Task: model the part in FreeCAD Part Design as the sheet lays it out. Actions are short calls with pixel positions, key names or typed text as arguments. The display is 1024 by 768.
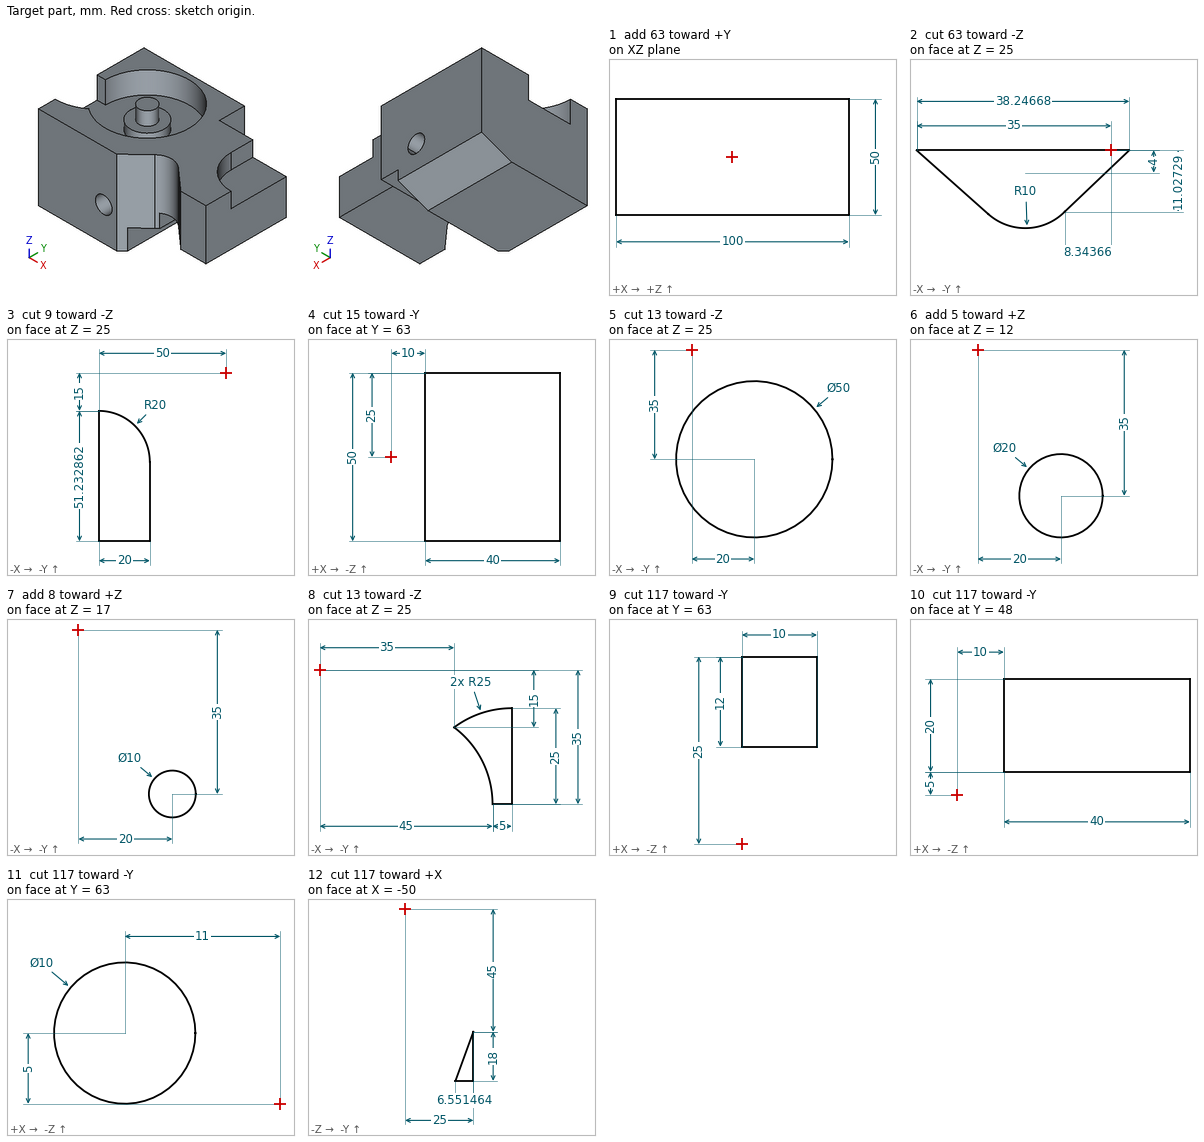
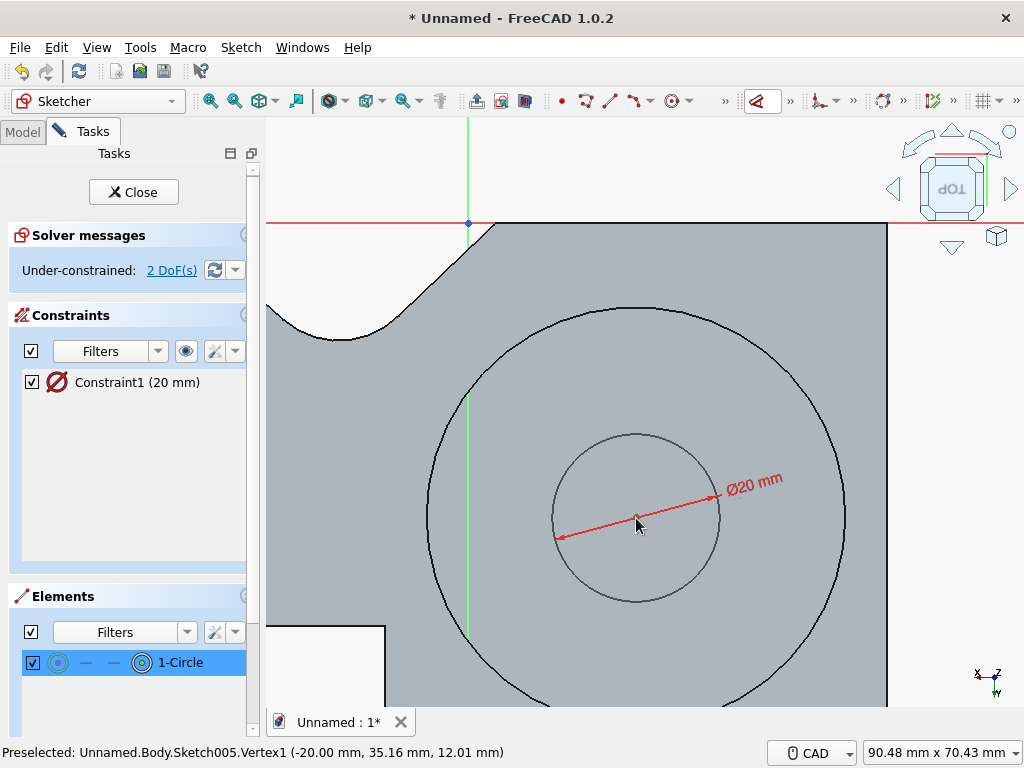
click(776, 102)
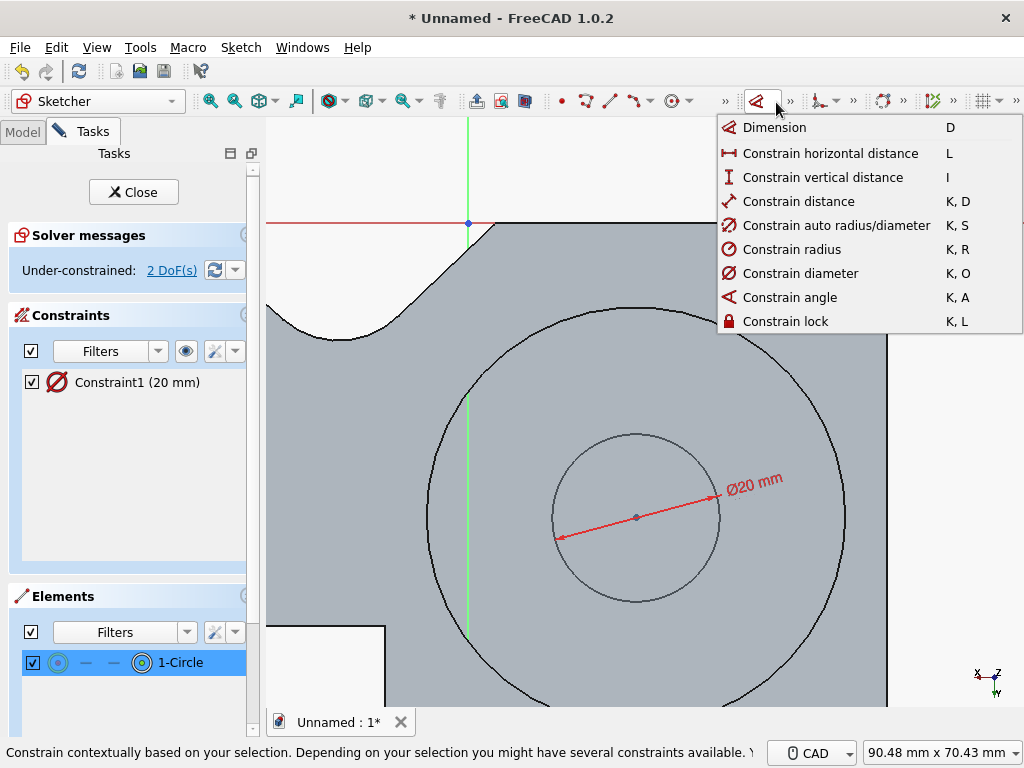
click(870, 153)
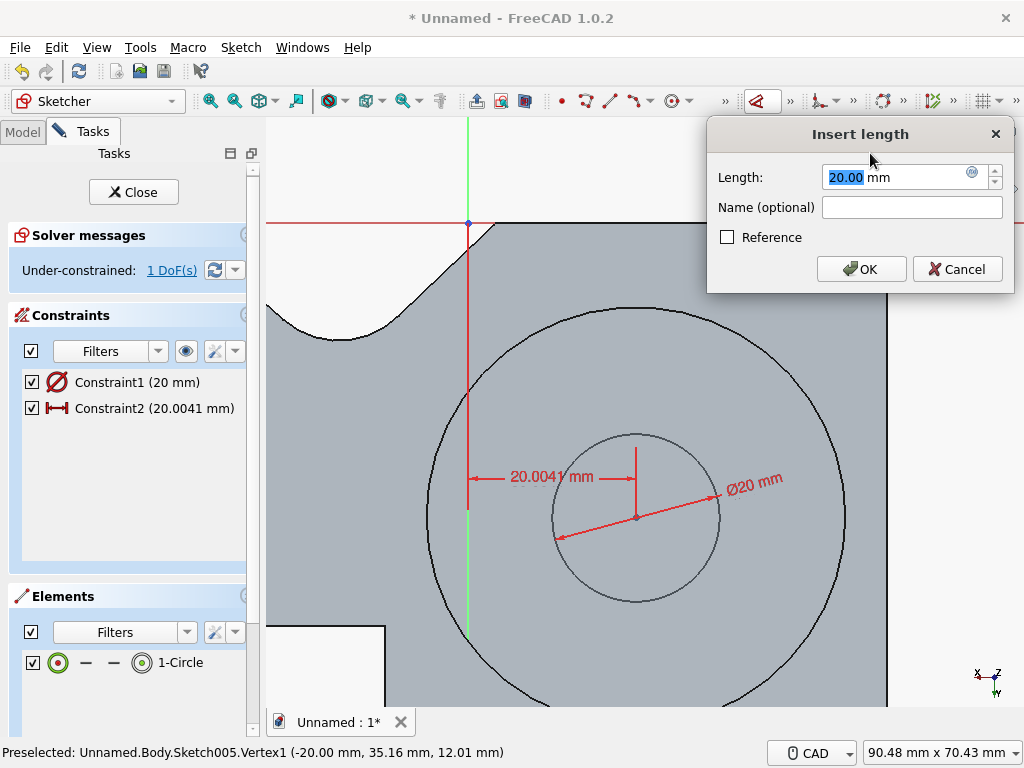
text(20)
key(Return)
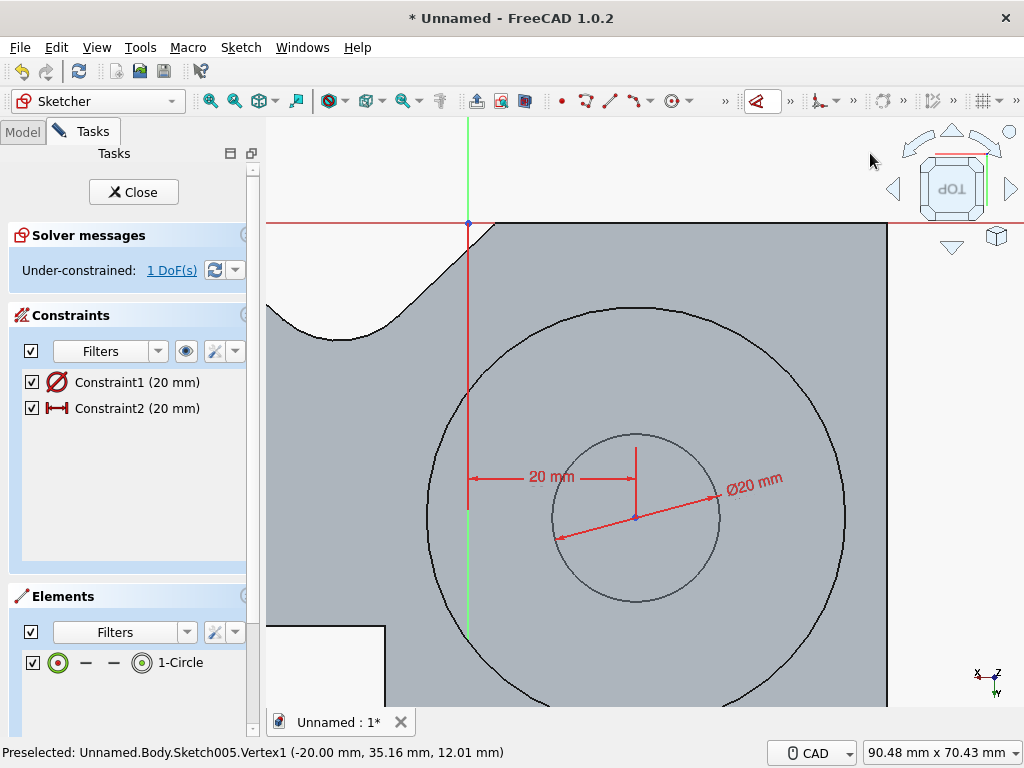
click(636, 518)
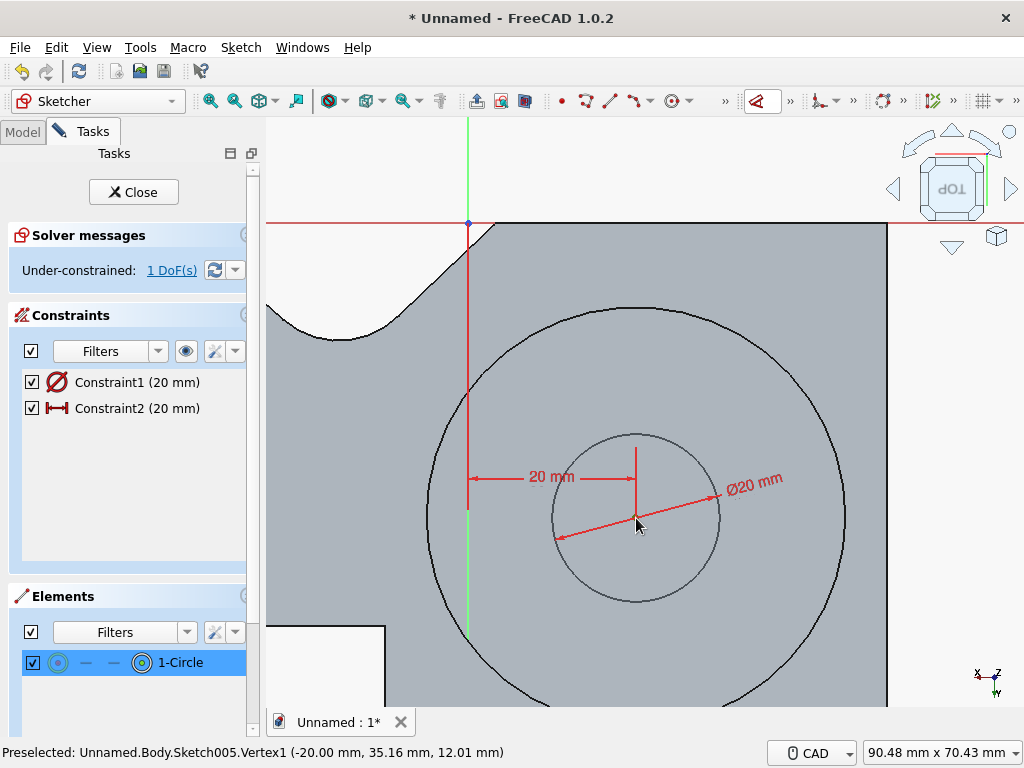
key(i)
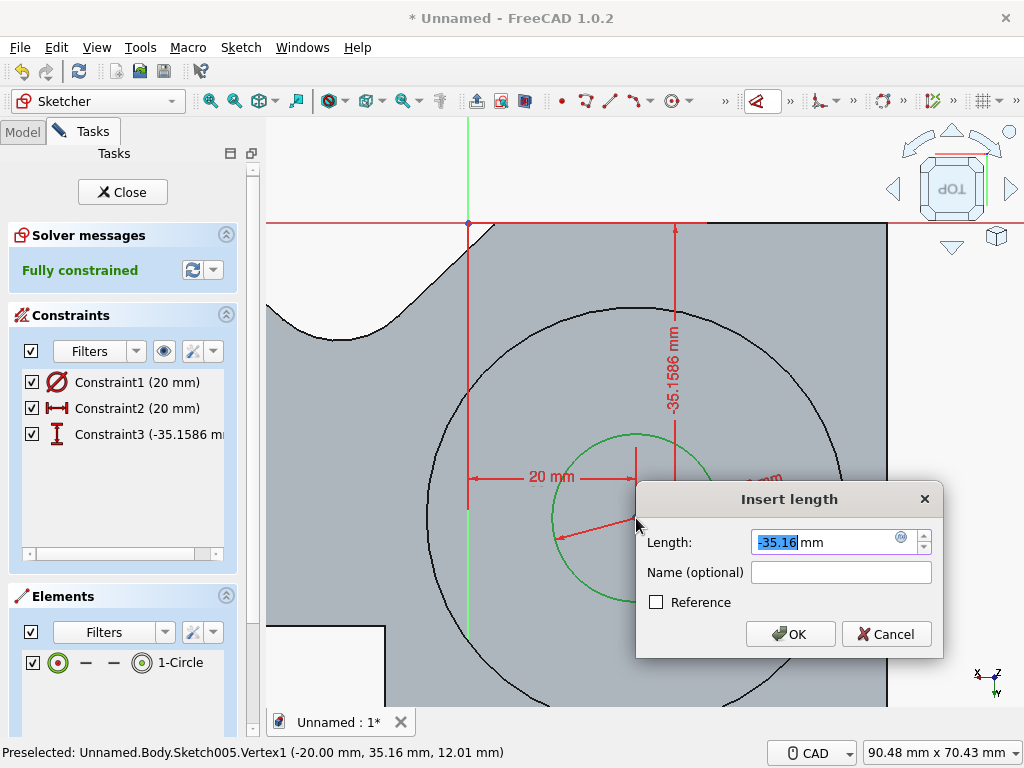
text(-35)
key(Return)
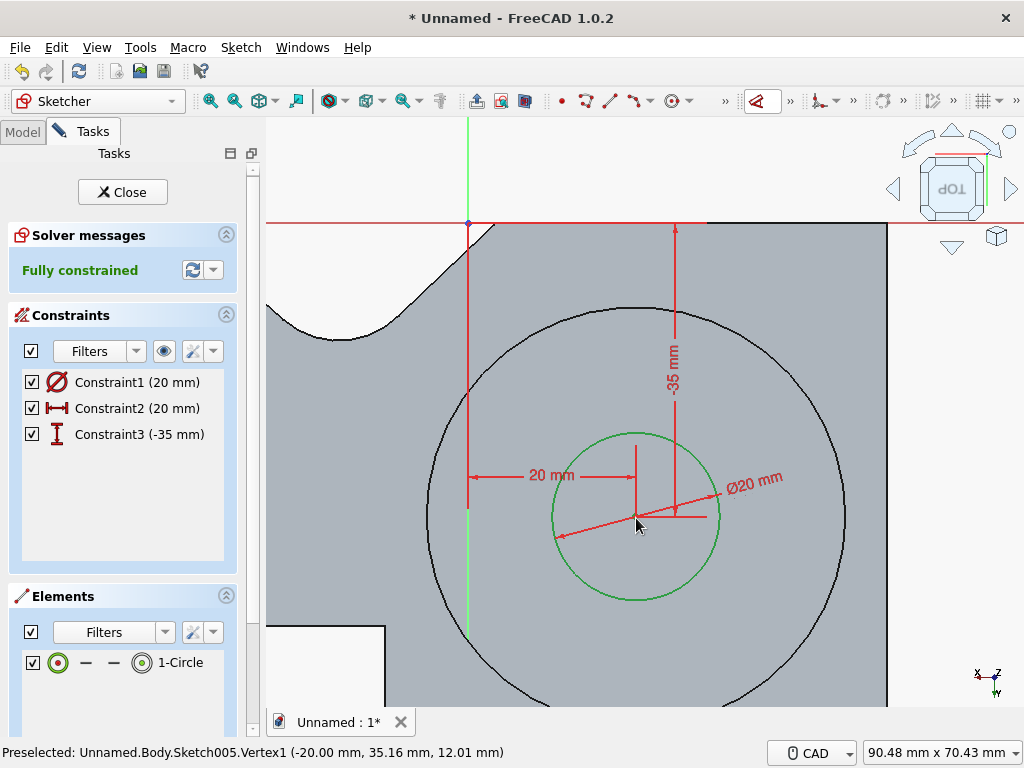
click(123, 192)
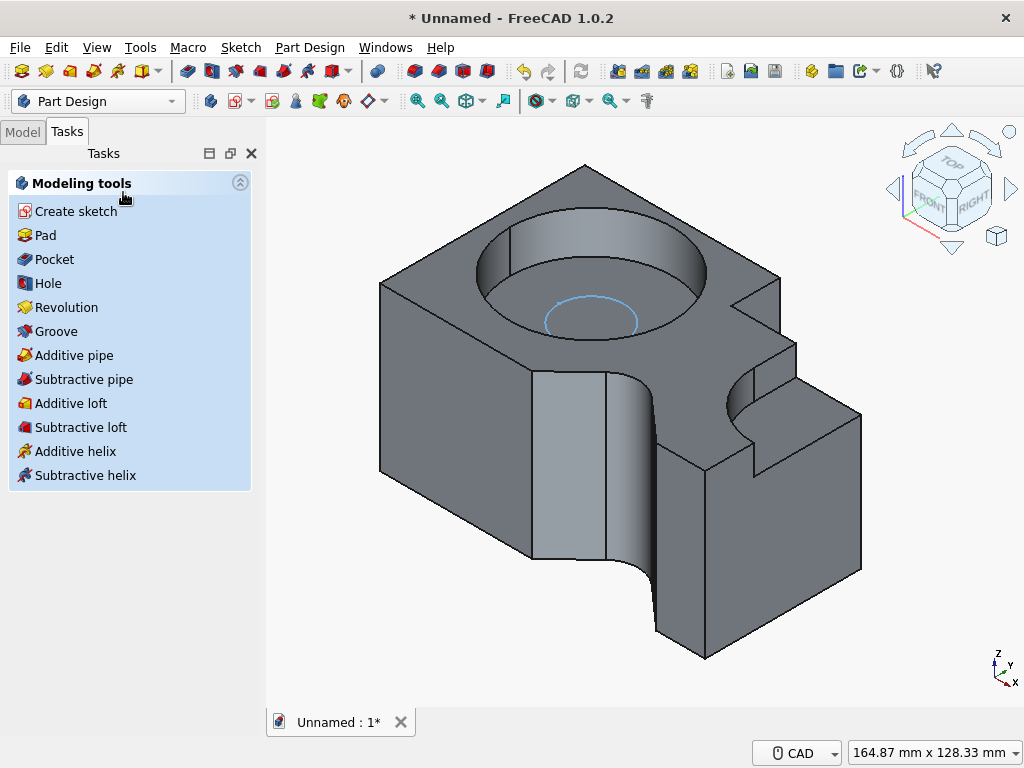
click(22, 72)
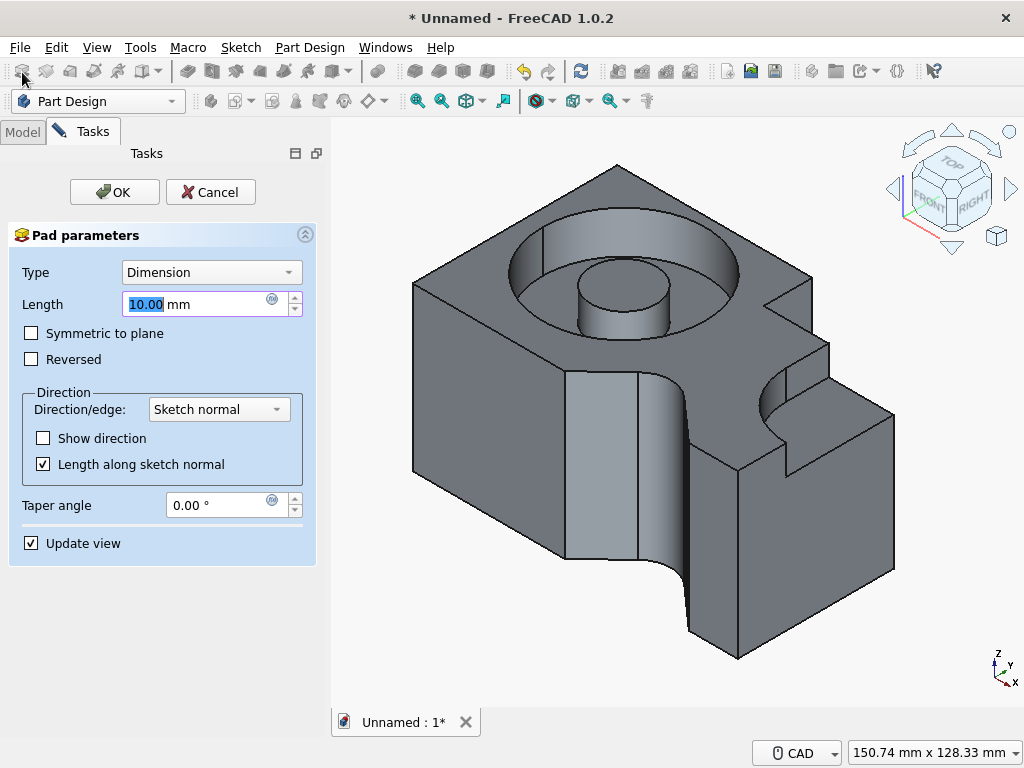
text(5)
key(Tab)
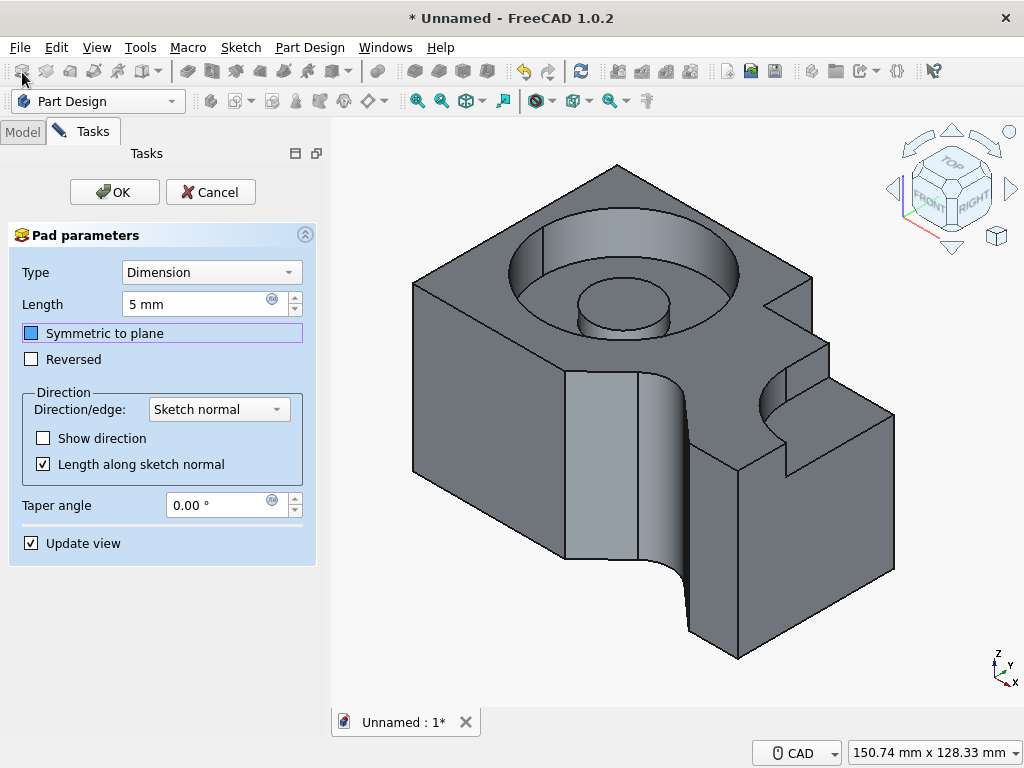
click(115, 192)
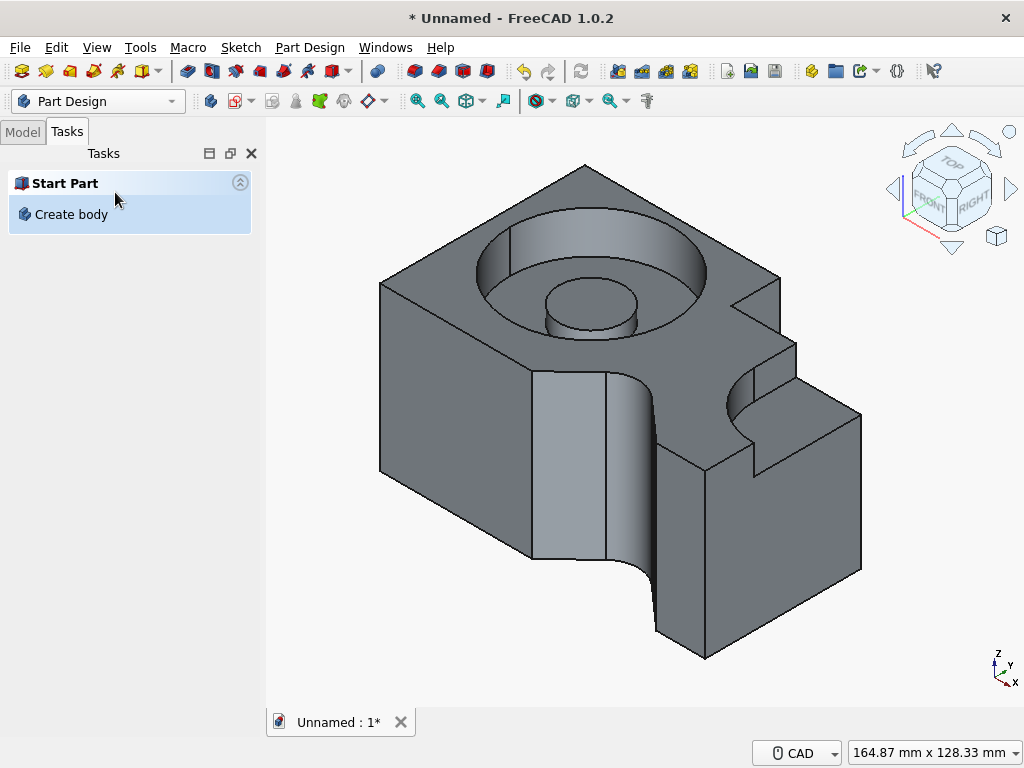
click(591, 303)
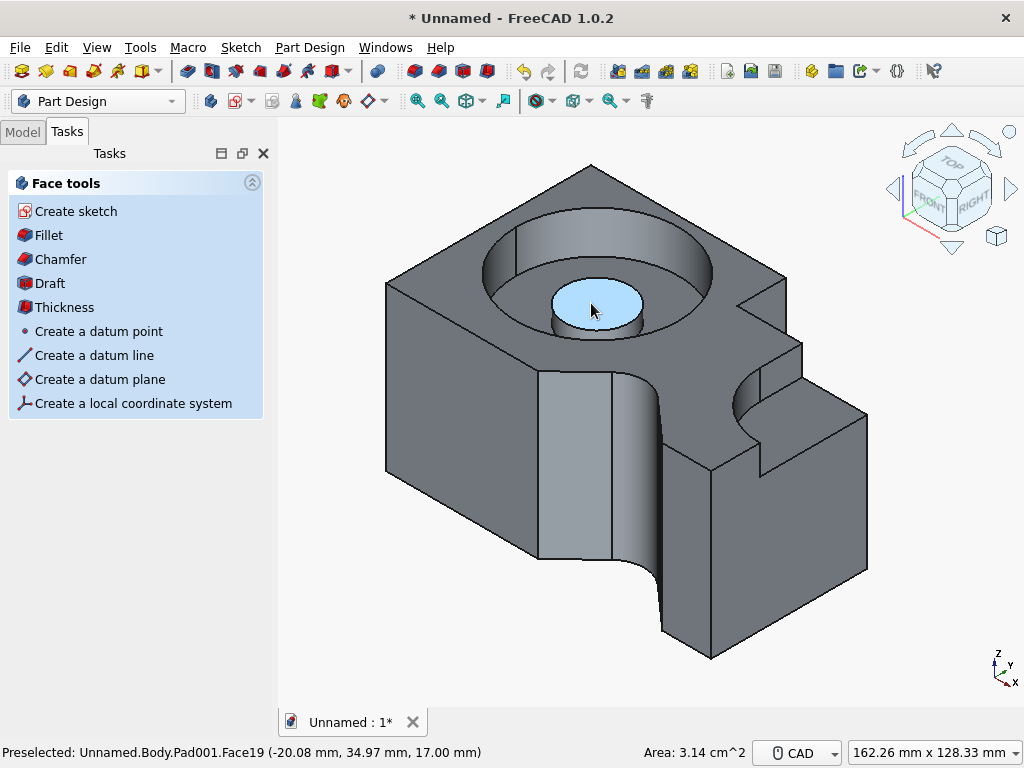
click(236, 102)